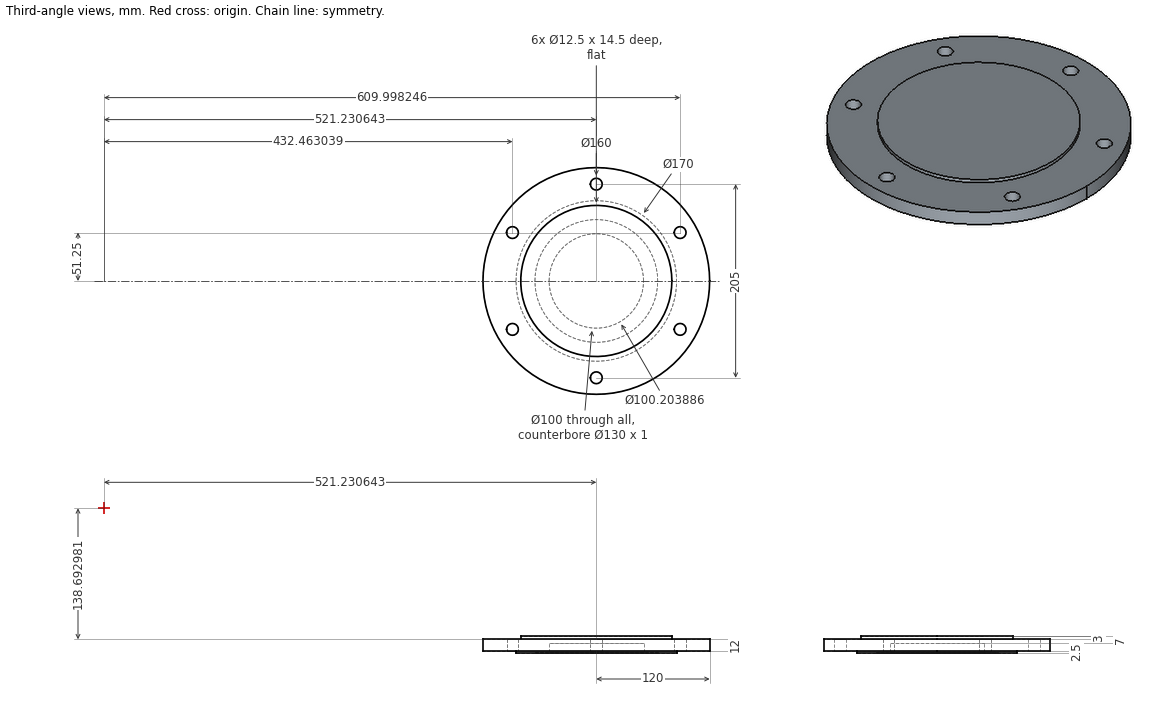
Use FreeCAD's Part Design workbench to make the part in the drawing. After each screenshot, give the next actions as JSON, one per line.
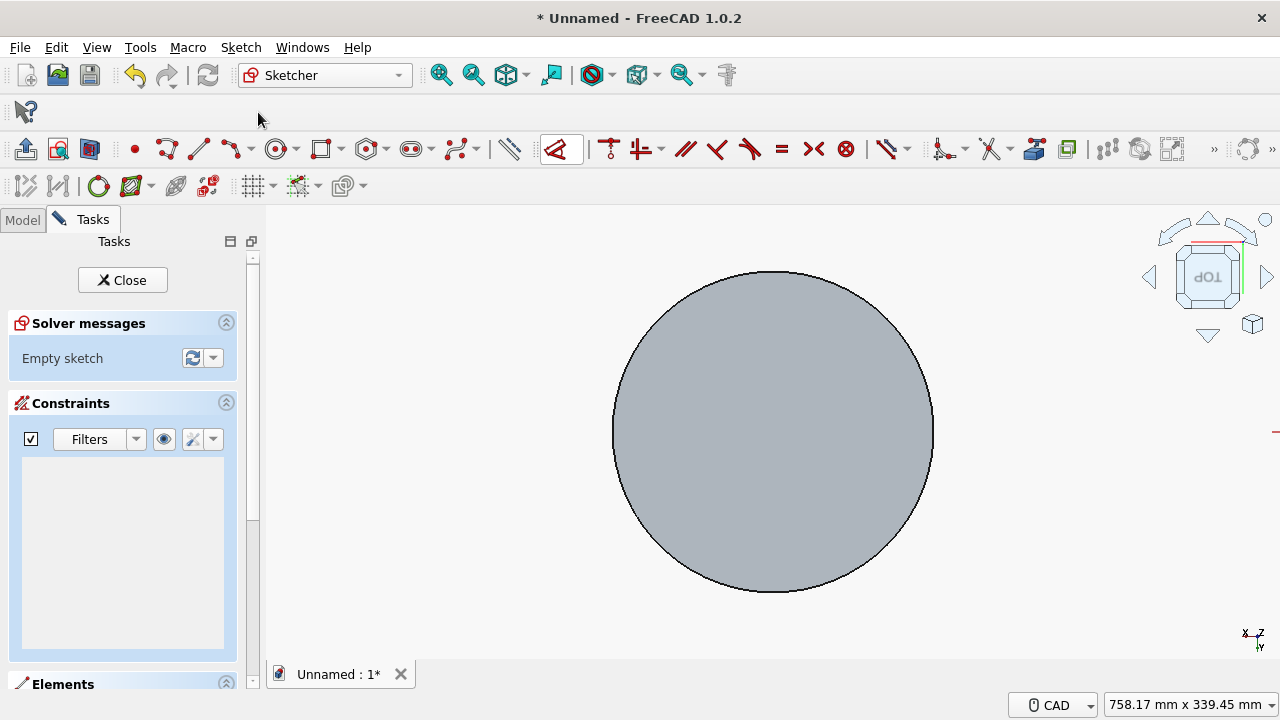
{"action": "key", "text": "g c"}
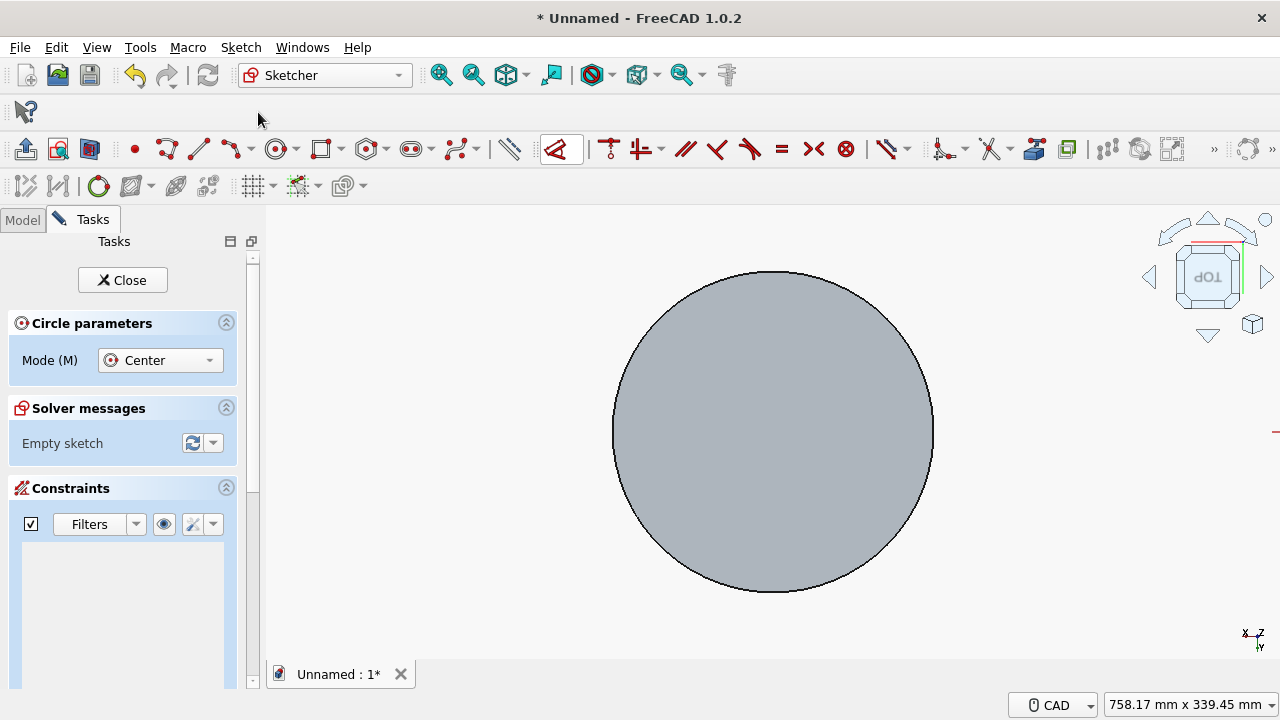
{"action": "left_click", "coordinate": [773, 432]}
{"action": "mouse_move", "coordinate": [849, 356]}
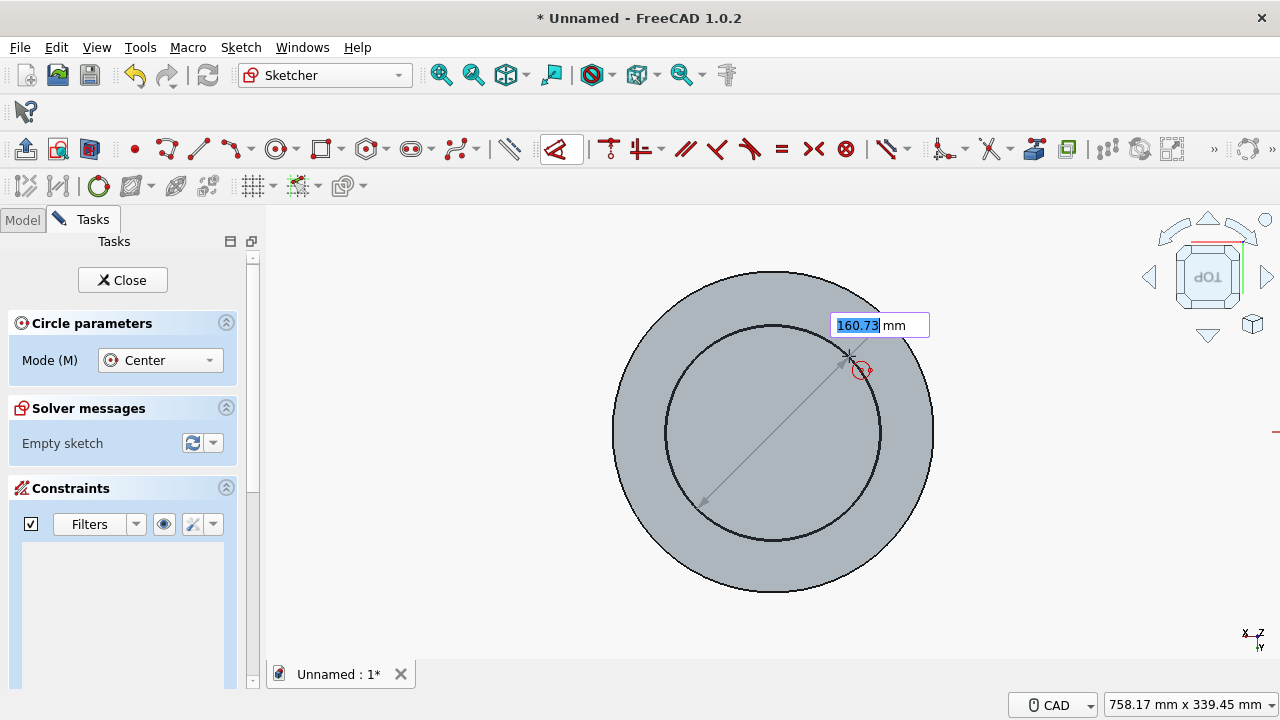
{"action": "type", "text": "160"}
{"action": "key", "text": "Return"}
{"action": "key", "text": "Escape"}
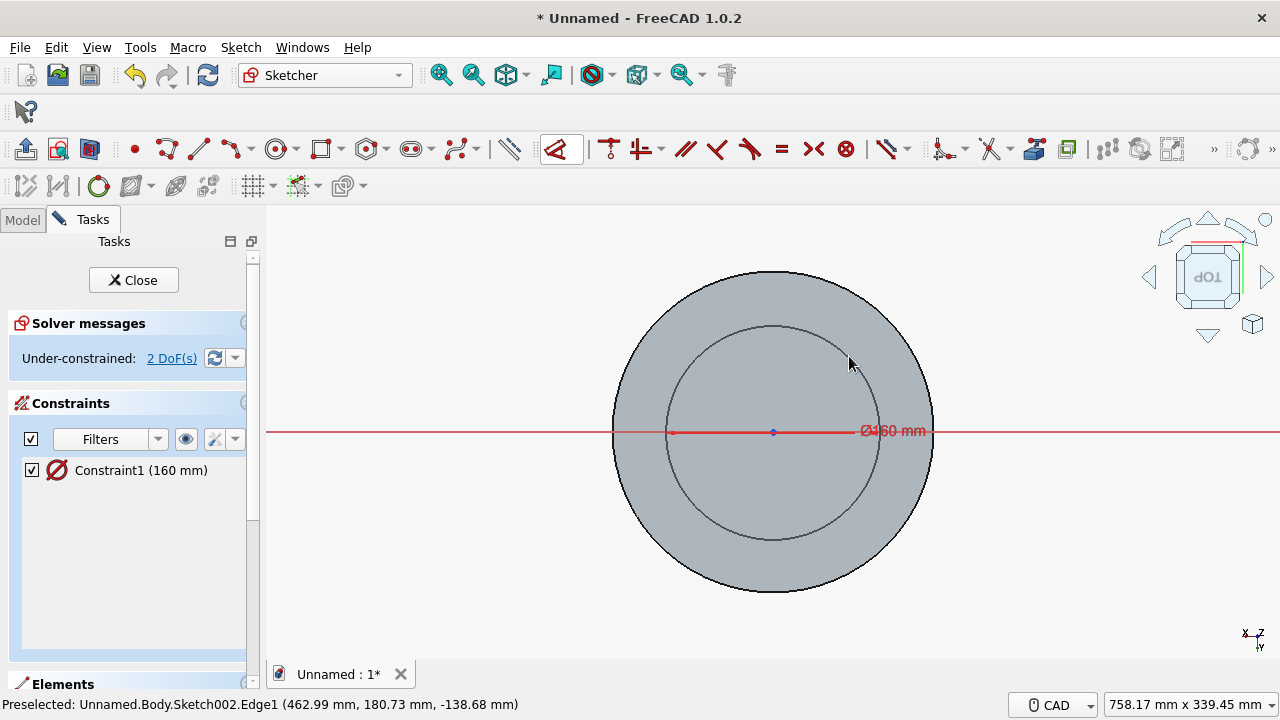
{"action": "left_click", "coordinate": [773, 433]}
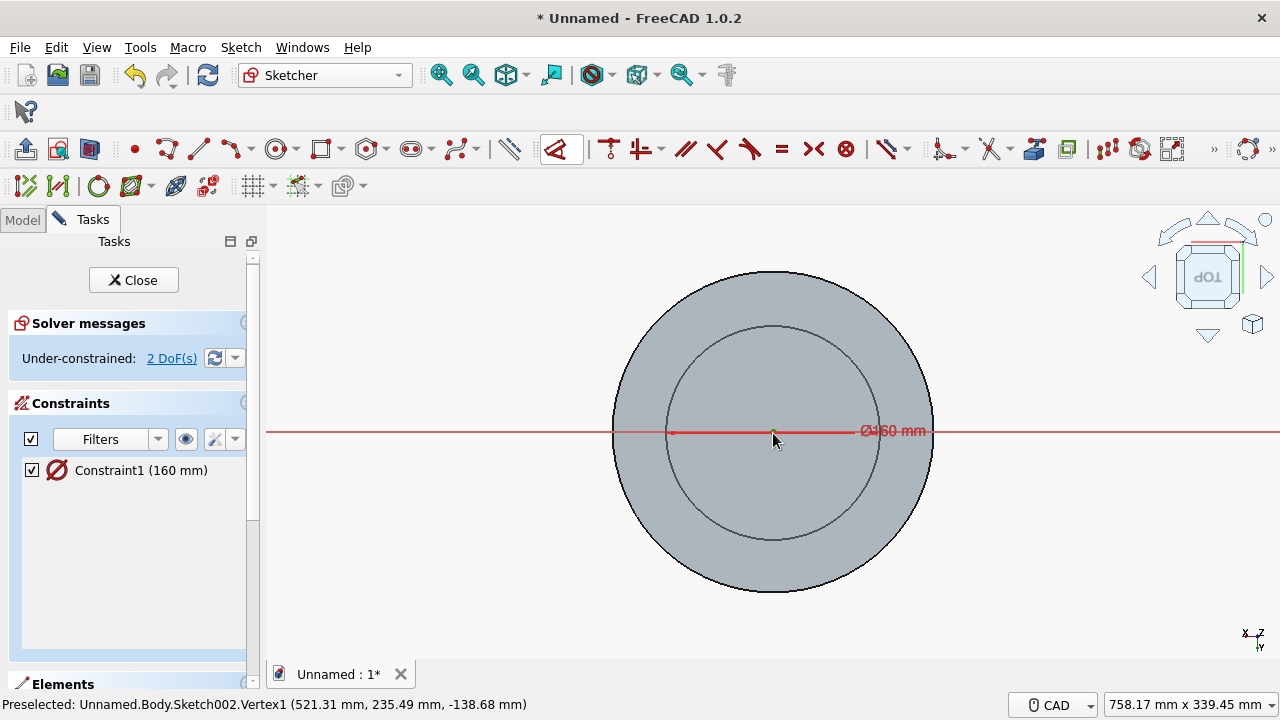
{"action": "left_click", "coordinate": [353, 432]}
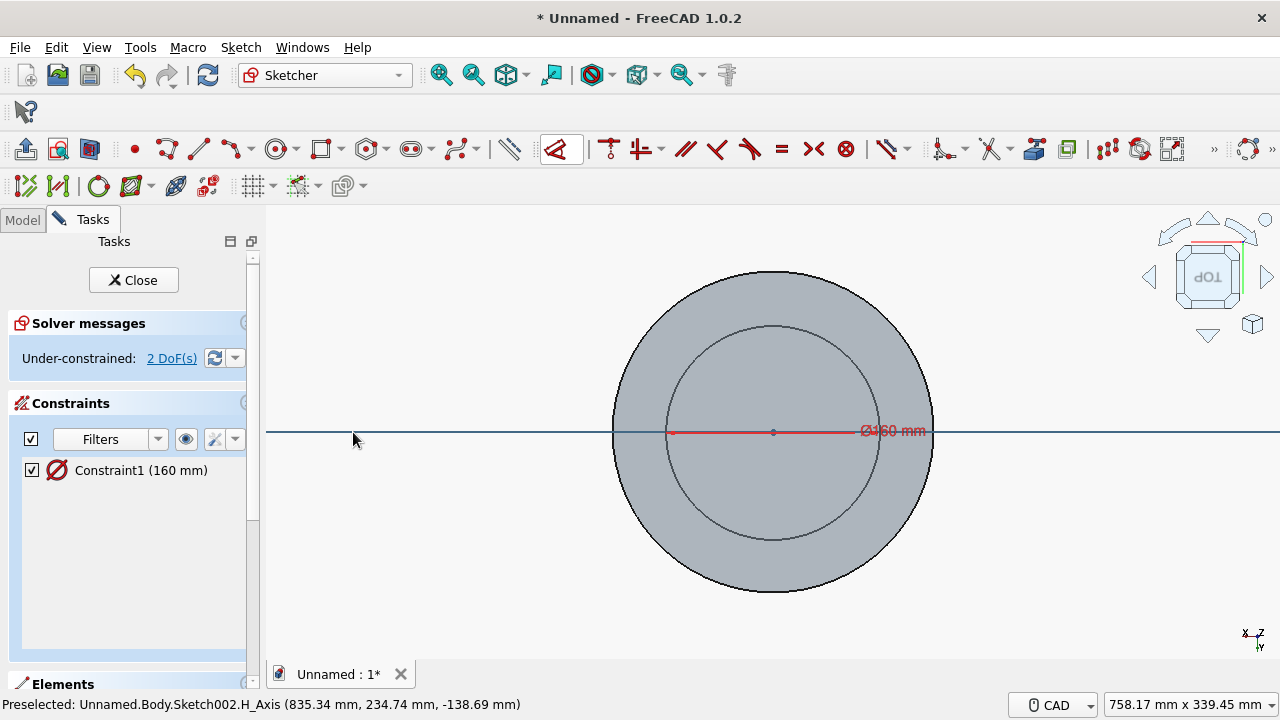
{"action": "left_click", "coordinate": [610, 150]}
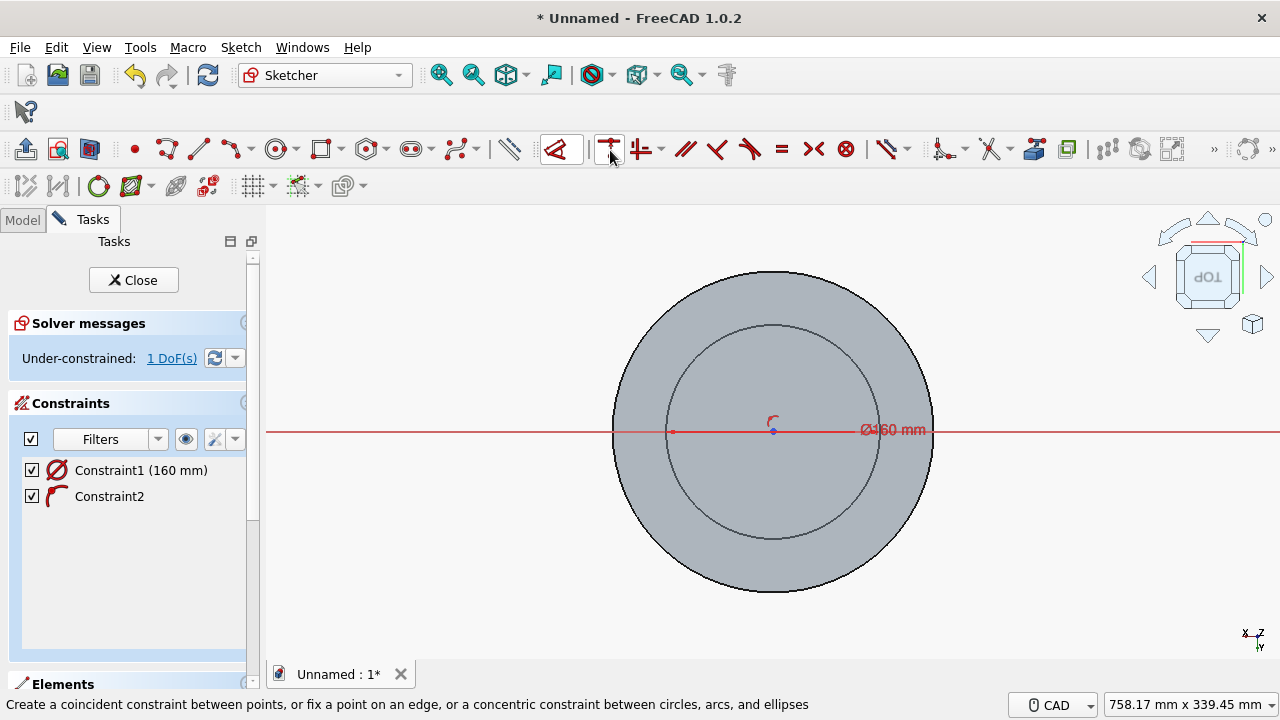
{"action": "key", "text": "d"}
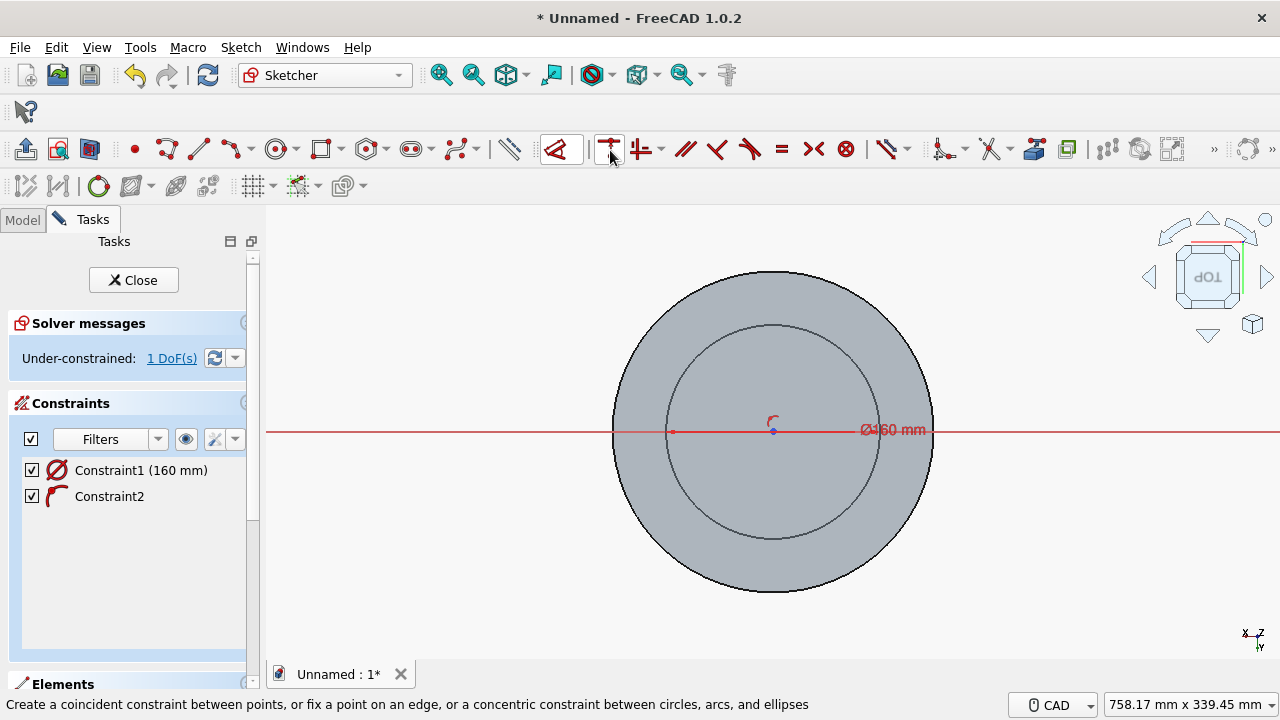
{"action": "left_click", "coordinate": [773, 432]}
{"action": "left_click", "coordinate": [944, 466]}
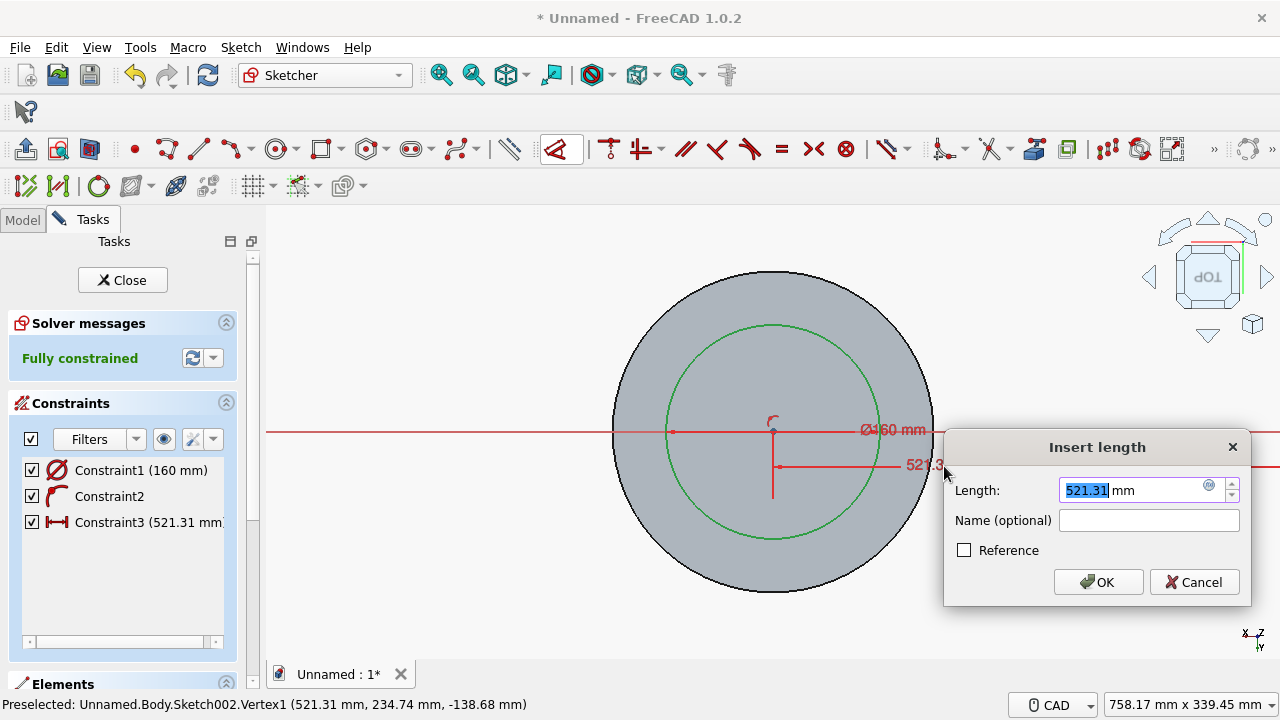
{"action": "type", "text": "521.230643"}
{"action": "key", "text": "Return"}
{"action": "key", "text": "Escape"}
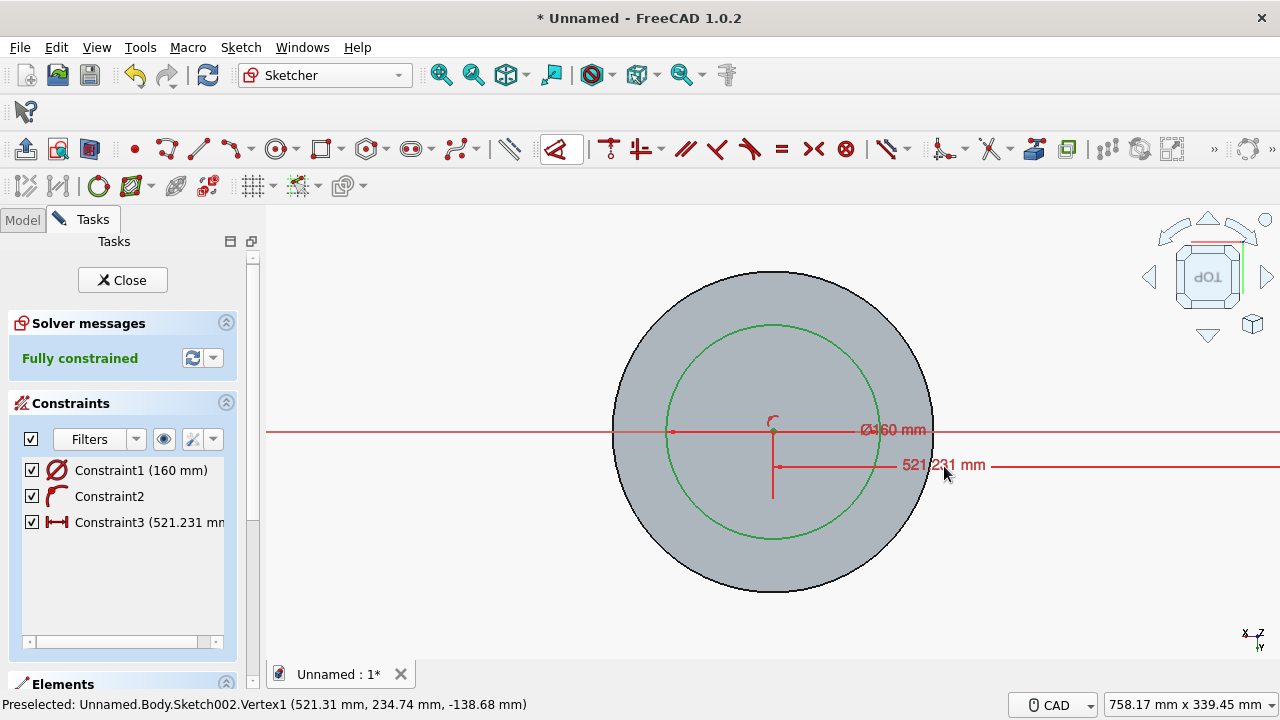
{"action": "left_click", "coordinate": [123, 280]}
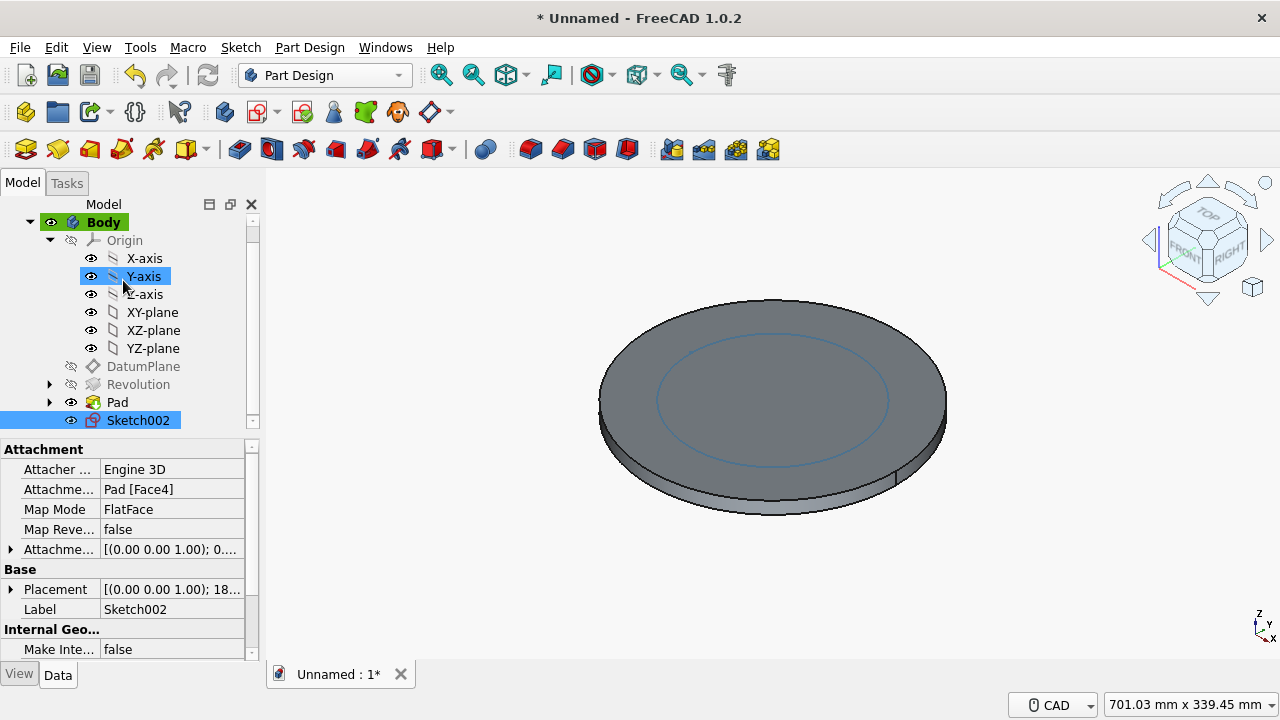
{"action": "left_click", "coordinate": [26, 150]}